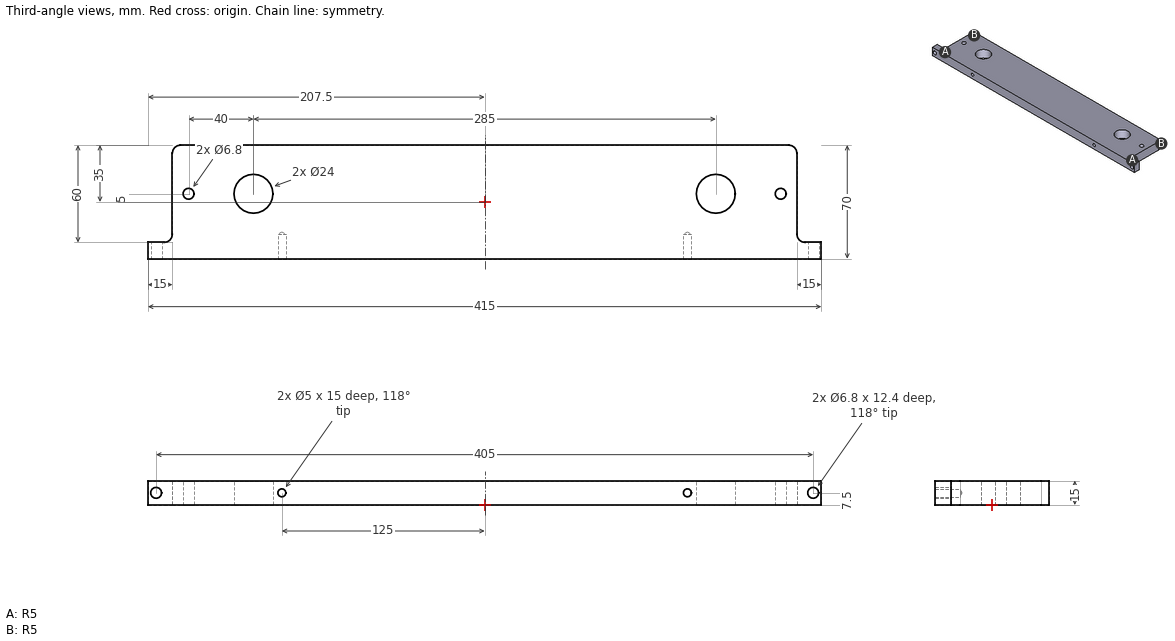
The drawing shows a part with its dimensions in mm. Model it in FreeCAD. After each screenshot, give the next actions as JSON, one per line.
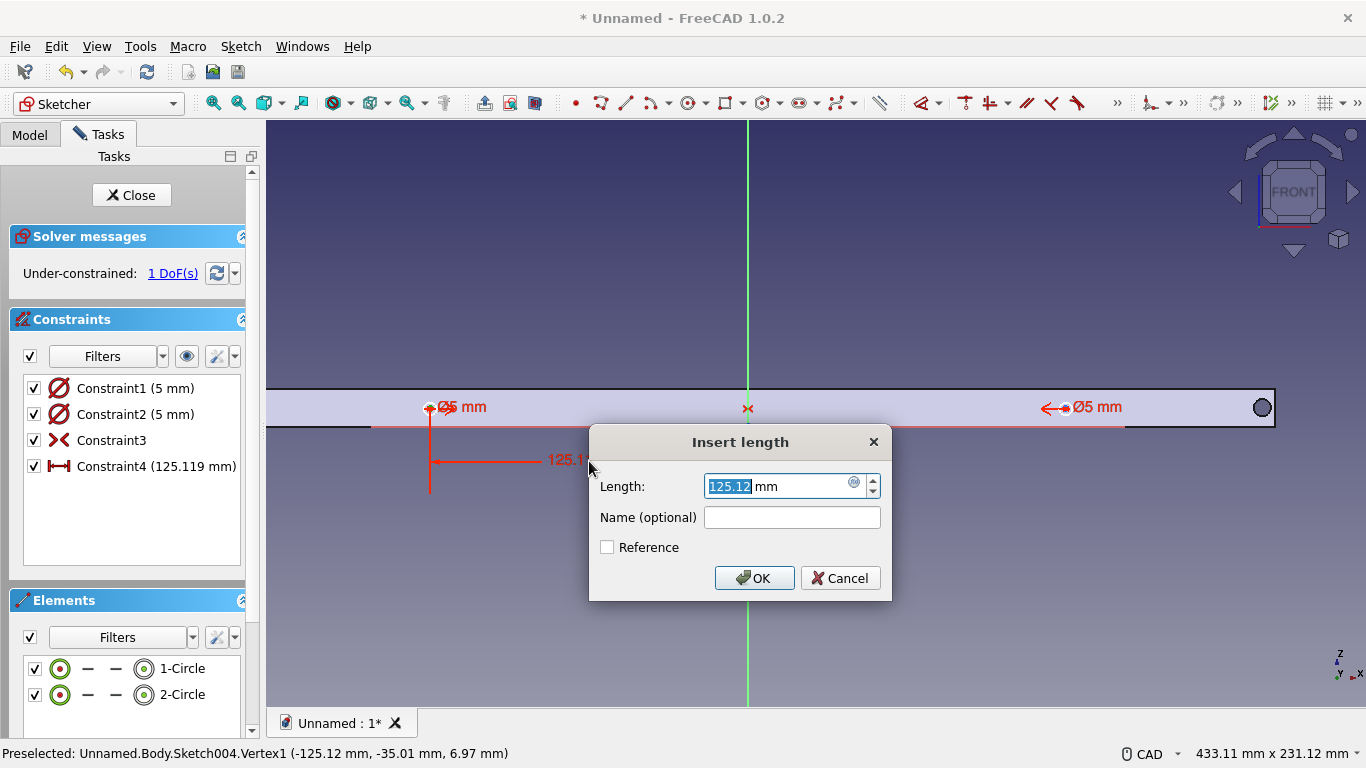
{"action": "type", "text": "125"}
{"action": "key", "text": "Return"}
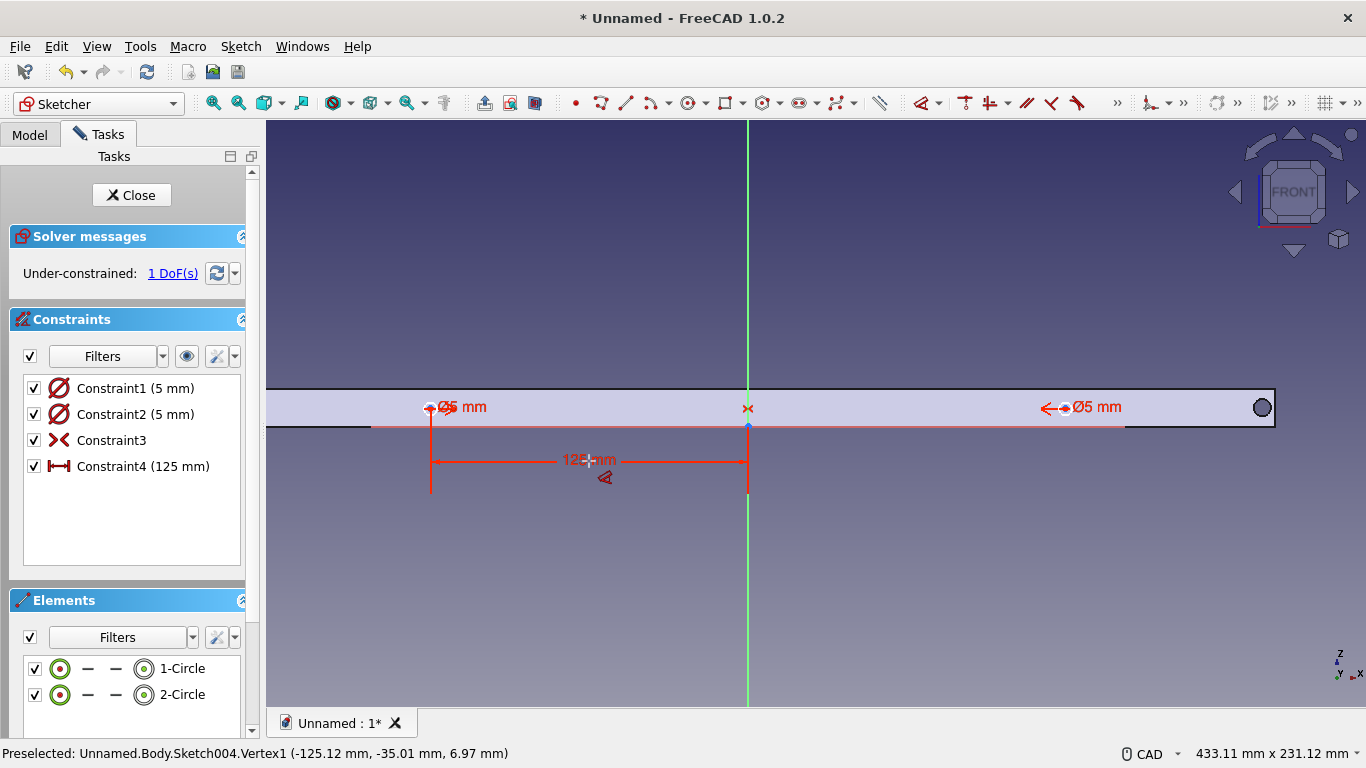
{"action": "scroll", "coordinate": [431, 409], "scroll_direction": "up", "scroll_amount": 4}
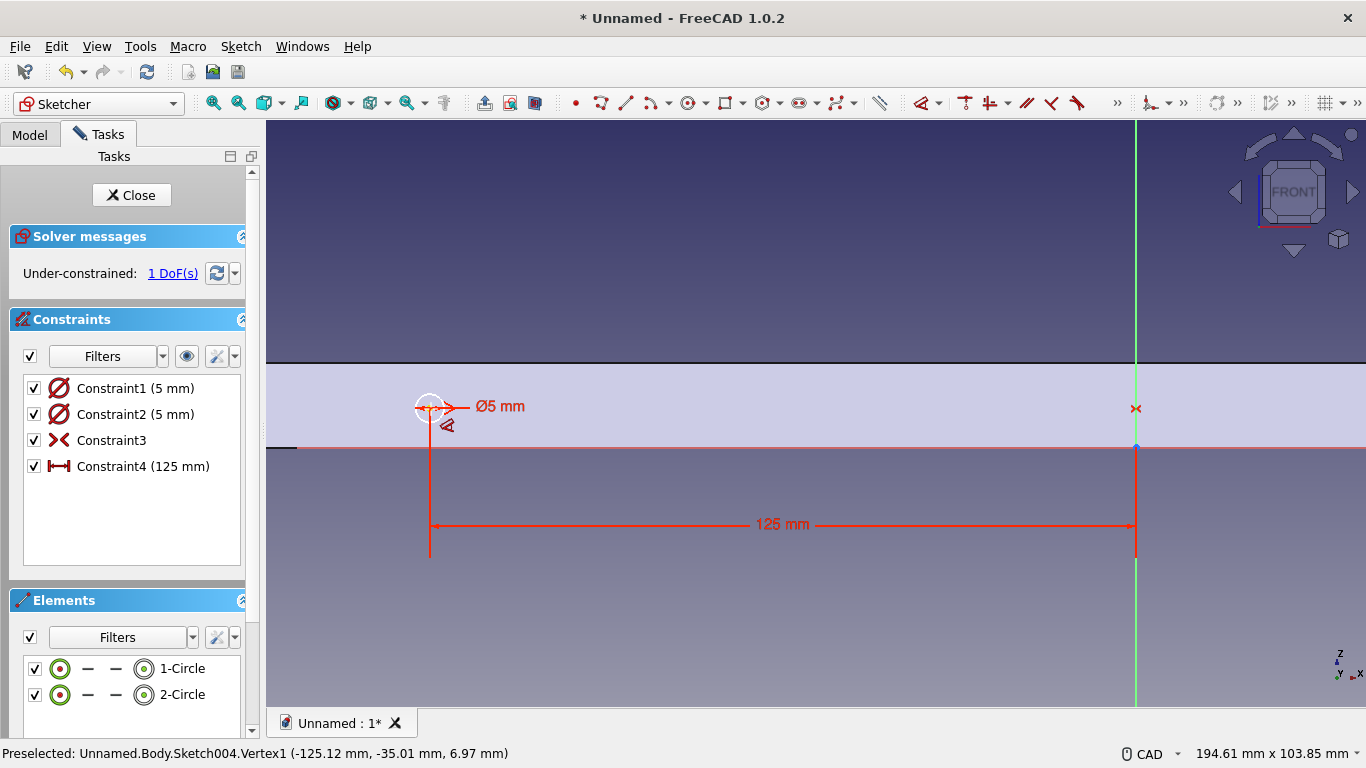
{"action": "left_click", "coordinate": [430, 408]}
{"action": "left_click", "coordinate": [396, 428]}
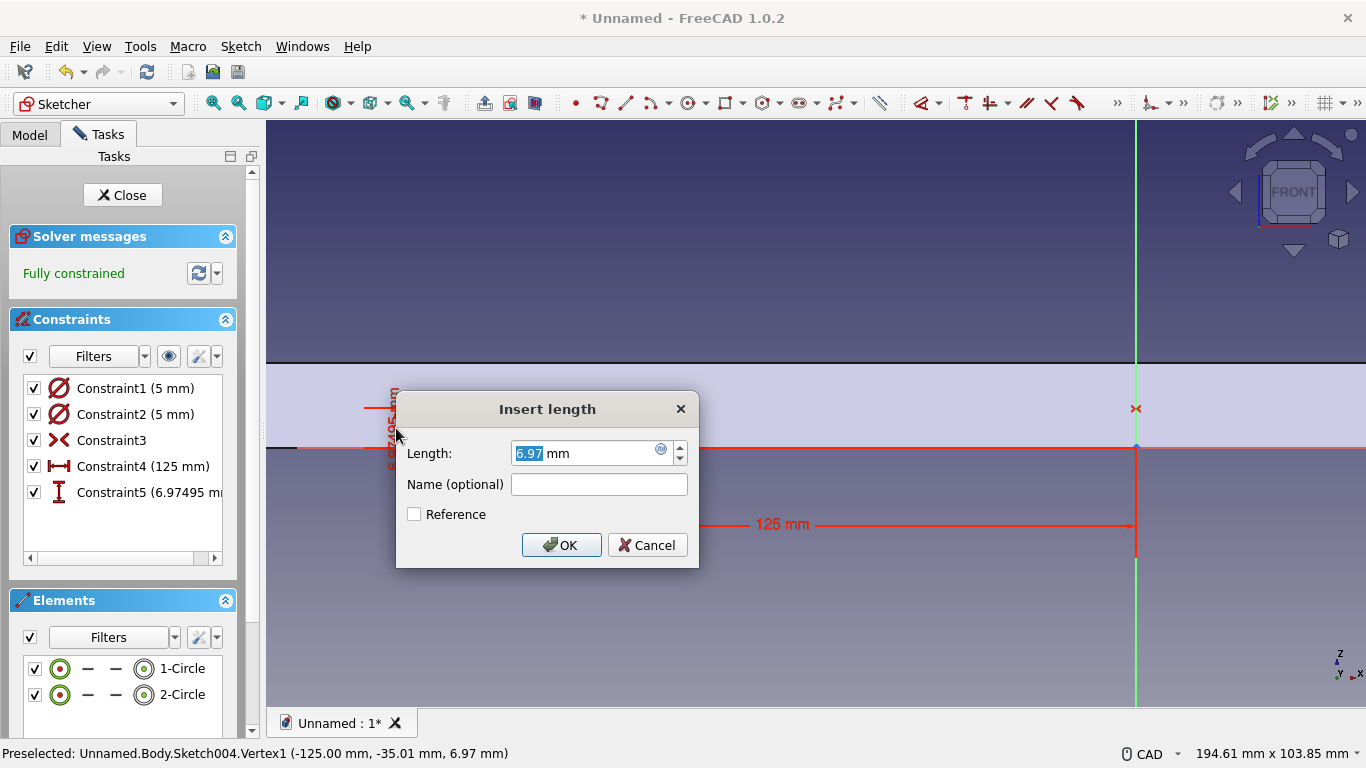
{"action": "type", "text": "7.5"}
{"action": "key", "text": "Return"}
{"action": "key", "text": "Escape"}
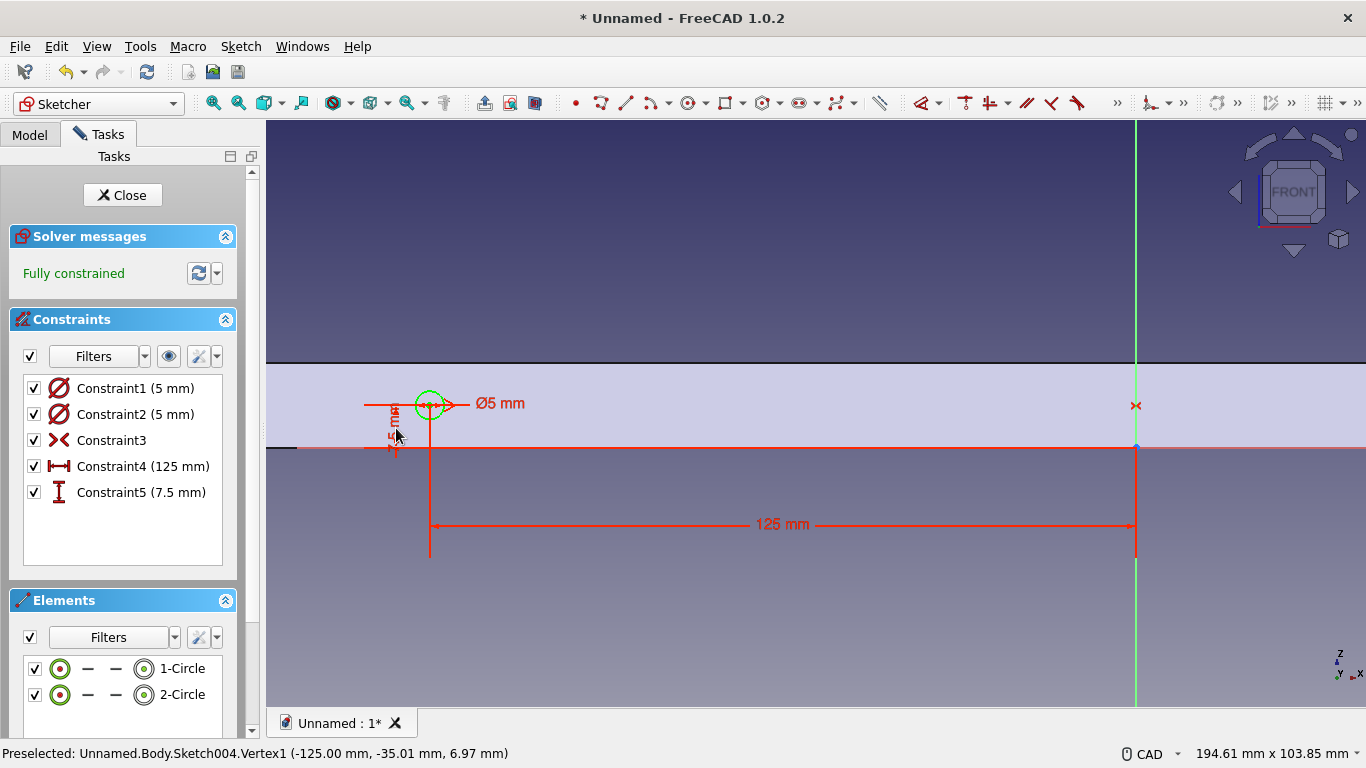
{"action": "left_click", "coordinate": [123, 195]}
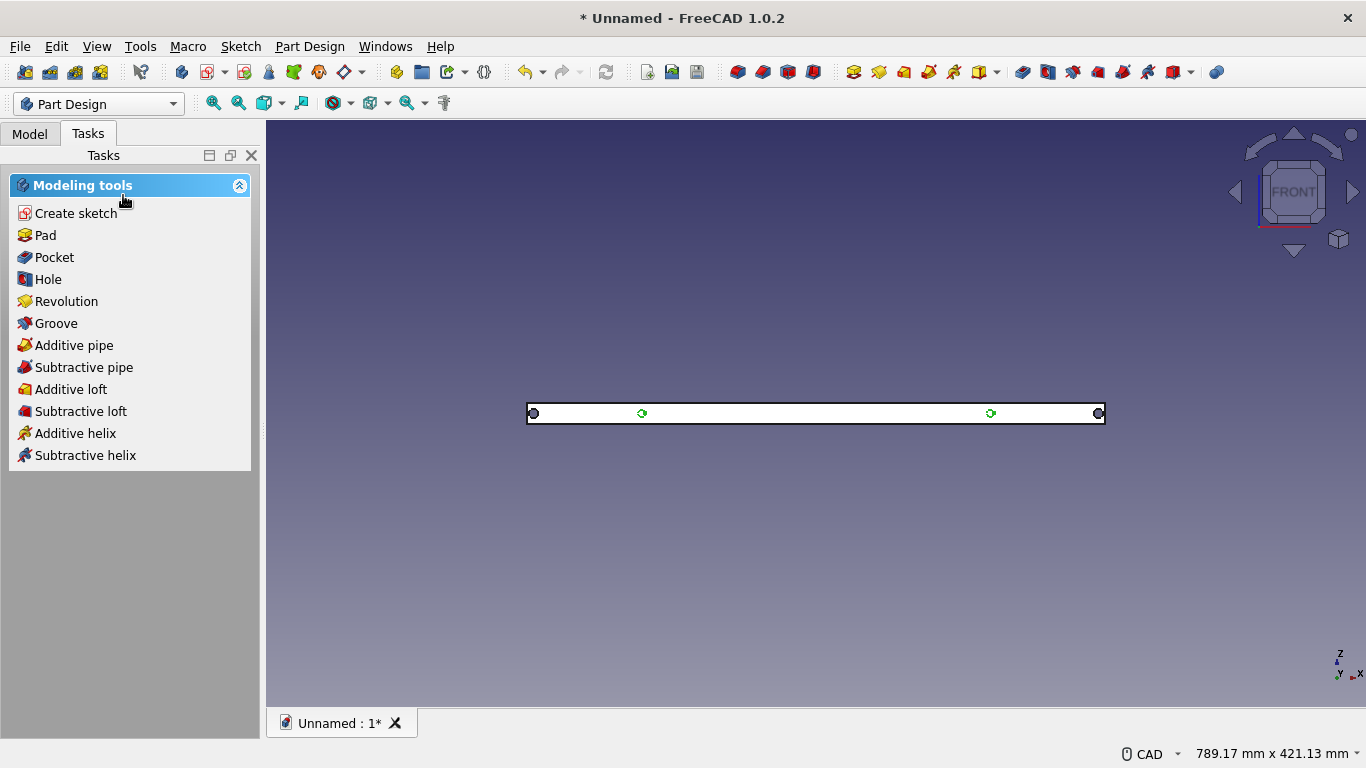
{"action": "left_click", "coordinate": [1048, 72]}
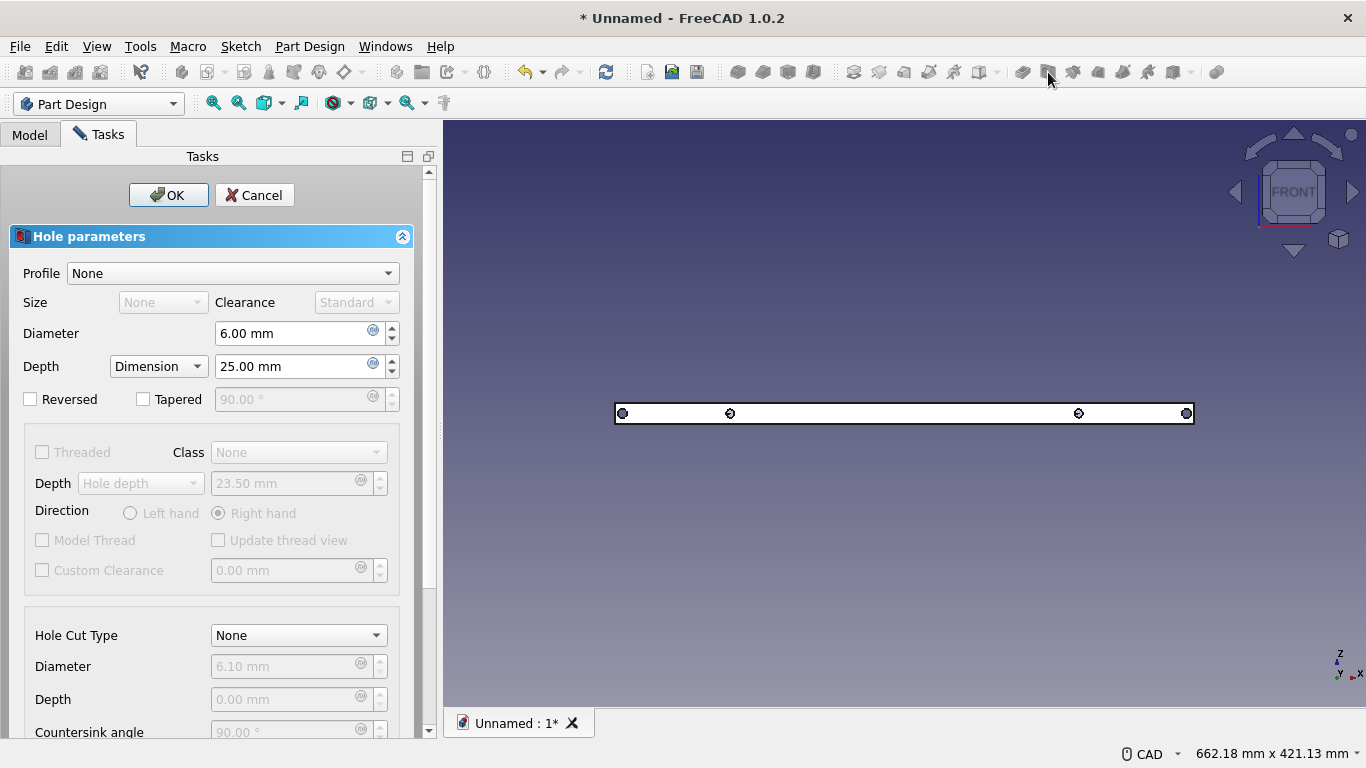
{"action": "triple_click", "coordinate": [300, 334]}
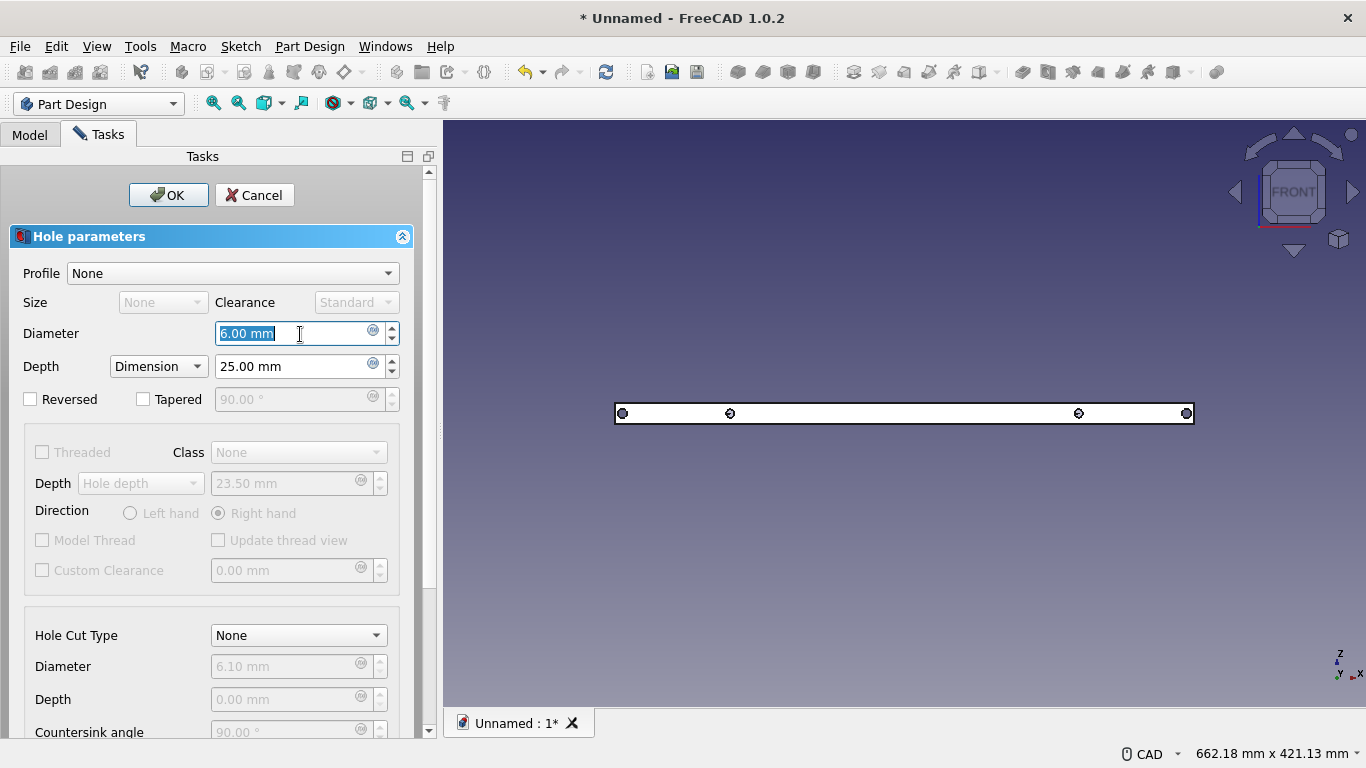
{"action": "type", "text": "5"}
{"action": "key", "text": "Tab"}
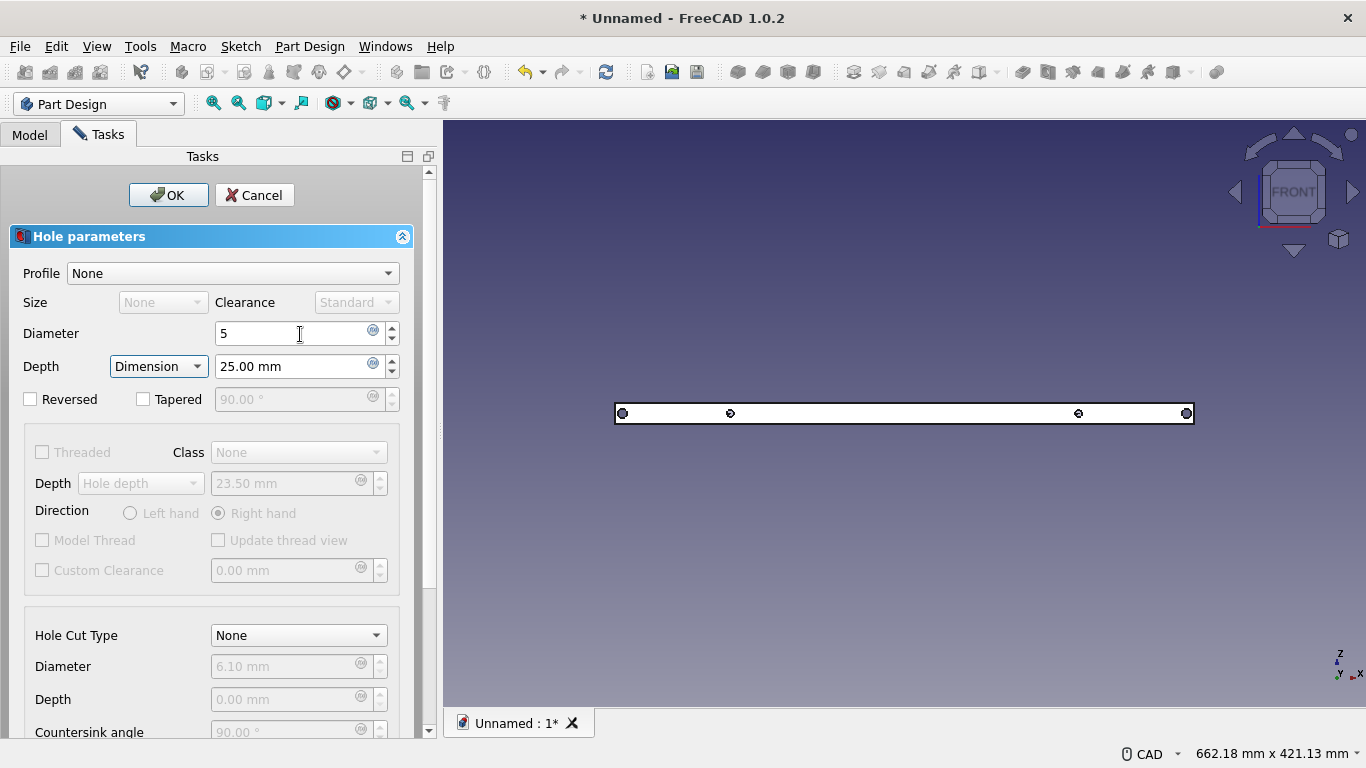
{"action": "triple_click", "coordinate": [300, 366]}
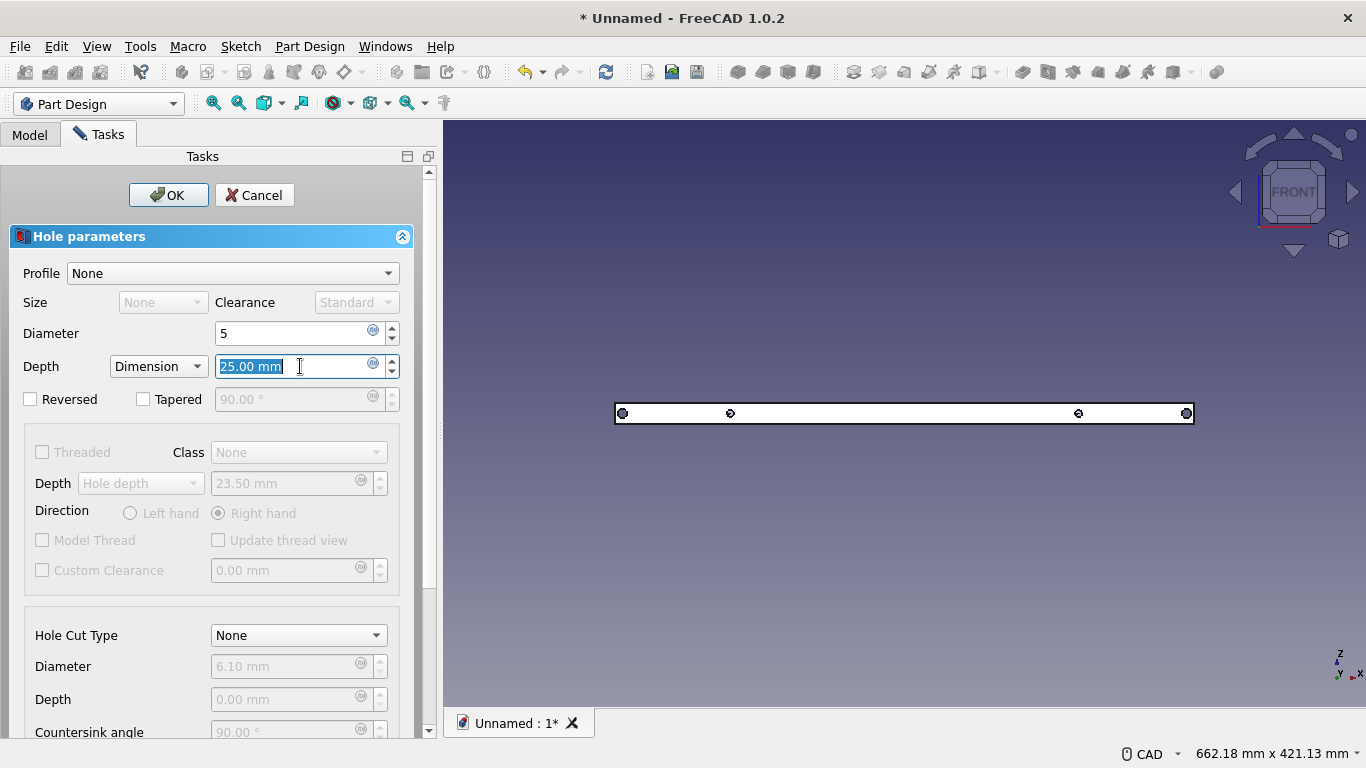
{"action": "type", "text": "15"}
{"action": "key", "text": "Tab"}